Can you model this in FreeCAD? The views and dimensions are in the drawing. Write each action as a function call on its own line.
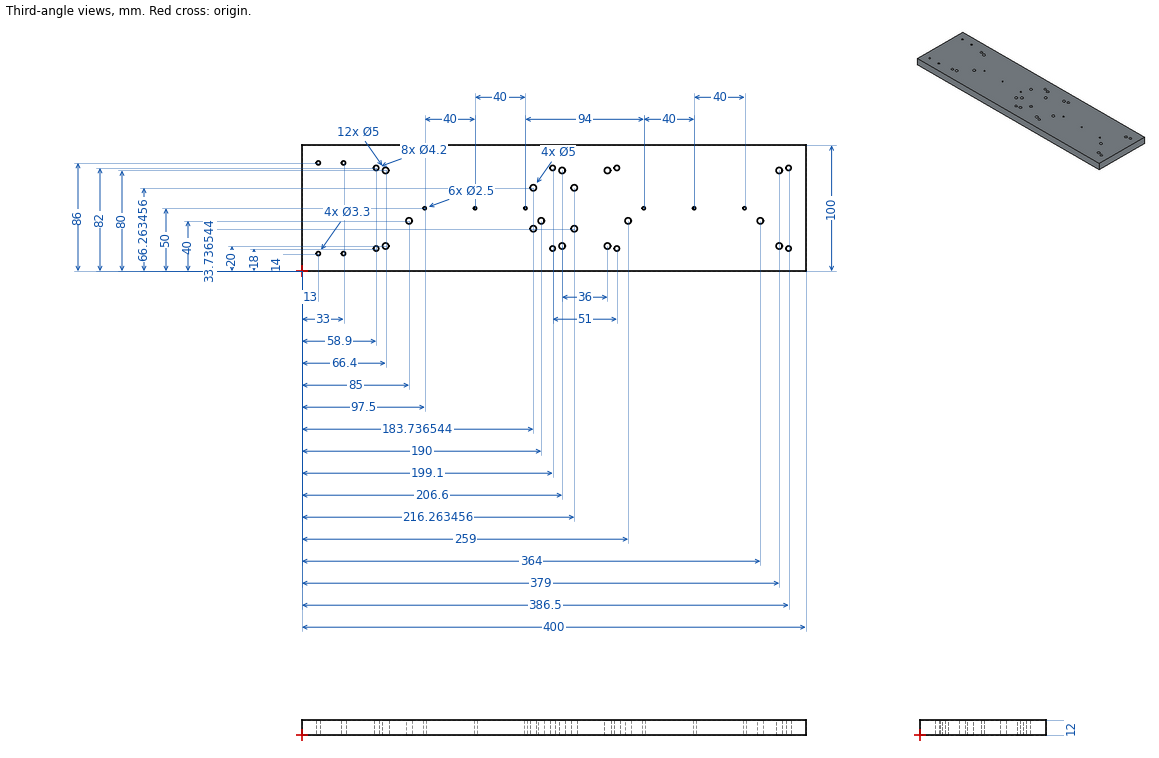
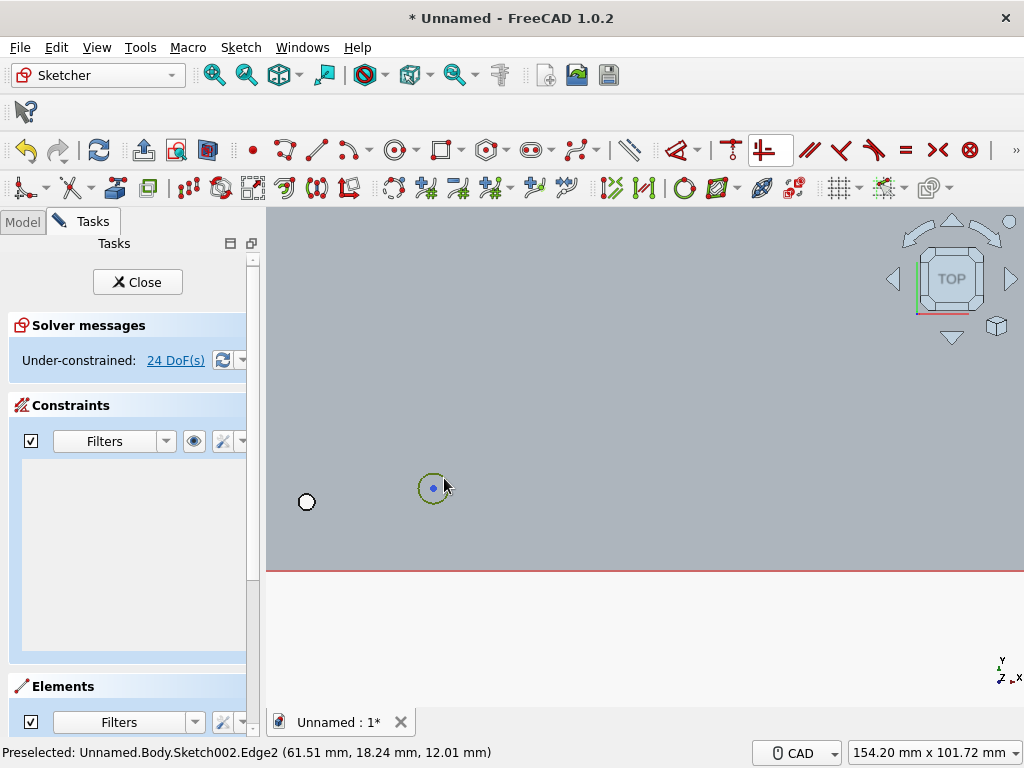
scroll(444, 480, down, 8)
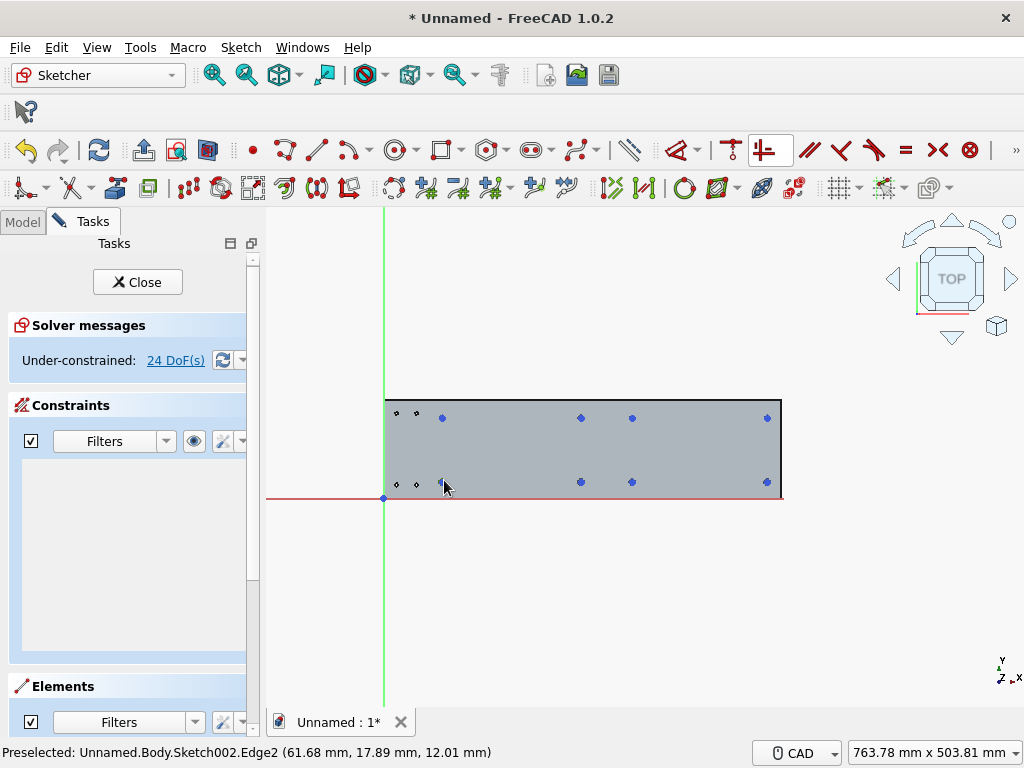
scroll(583, 416, up, 9)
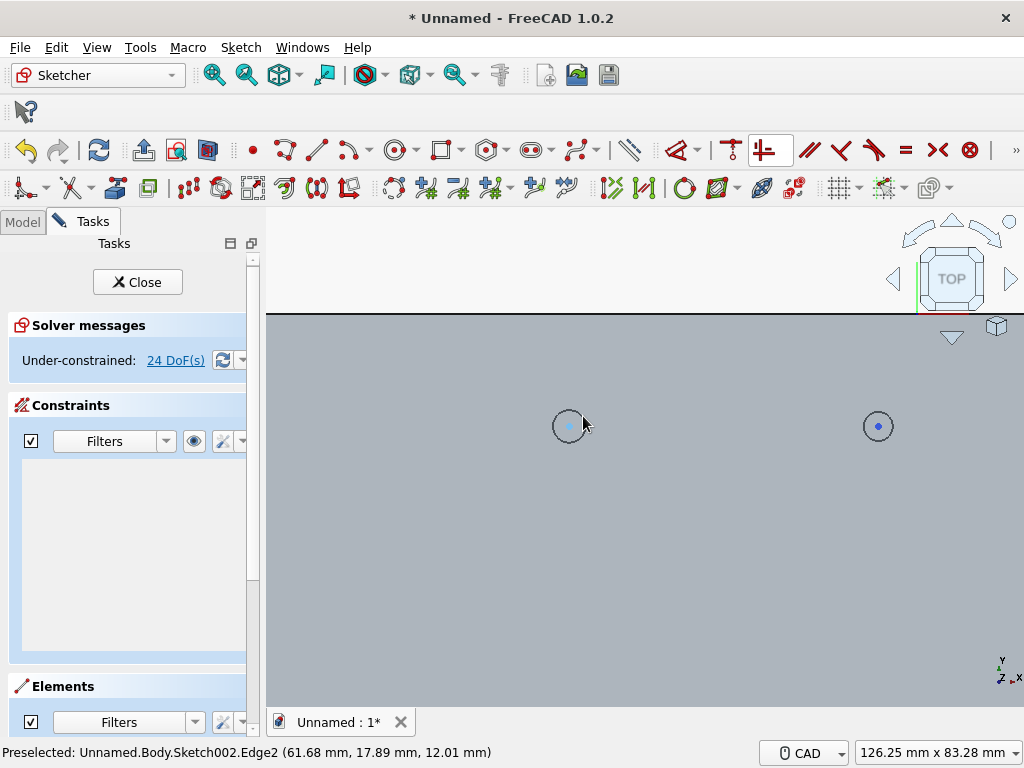
click(581, 415)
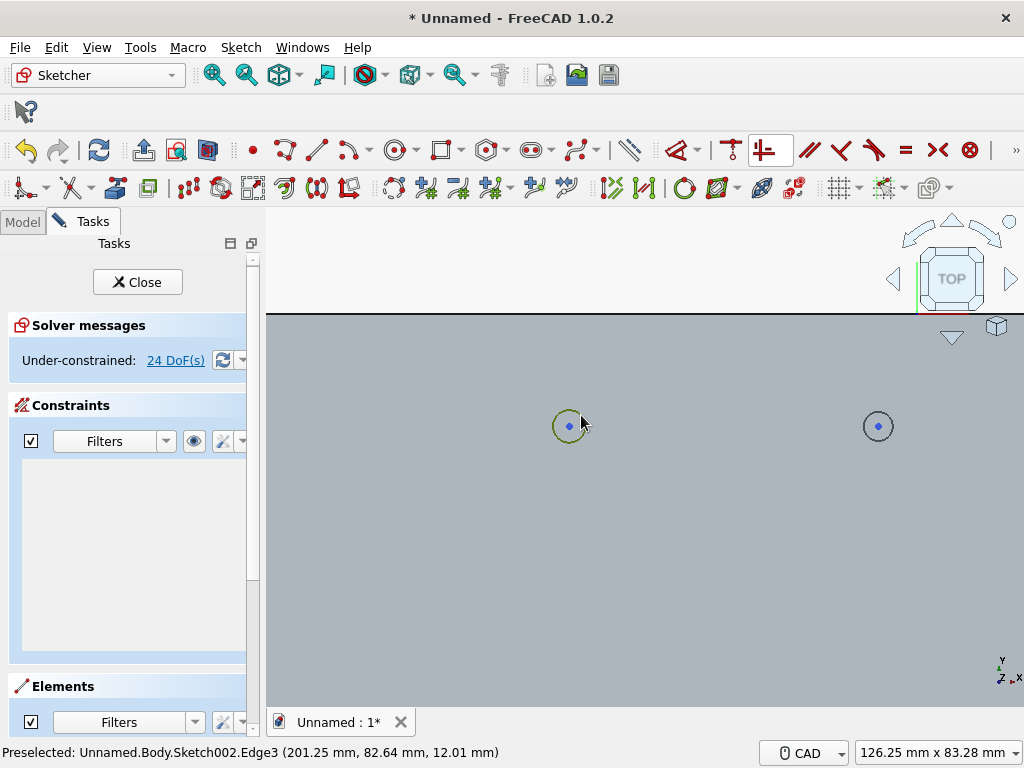
scroll(583, 416, down, 9)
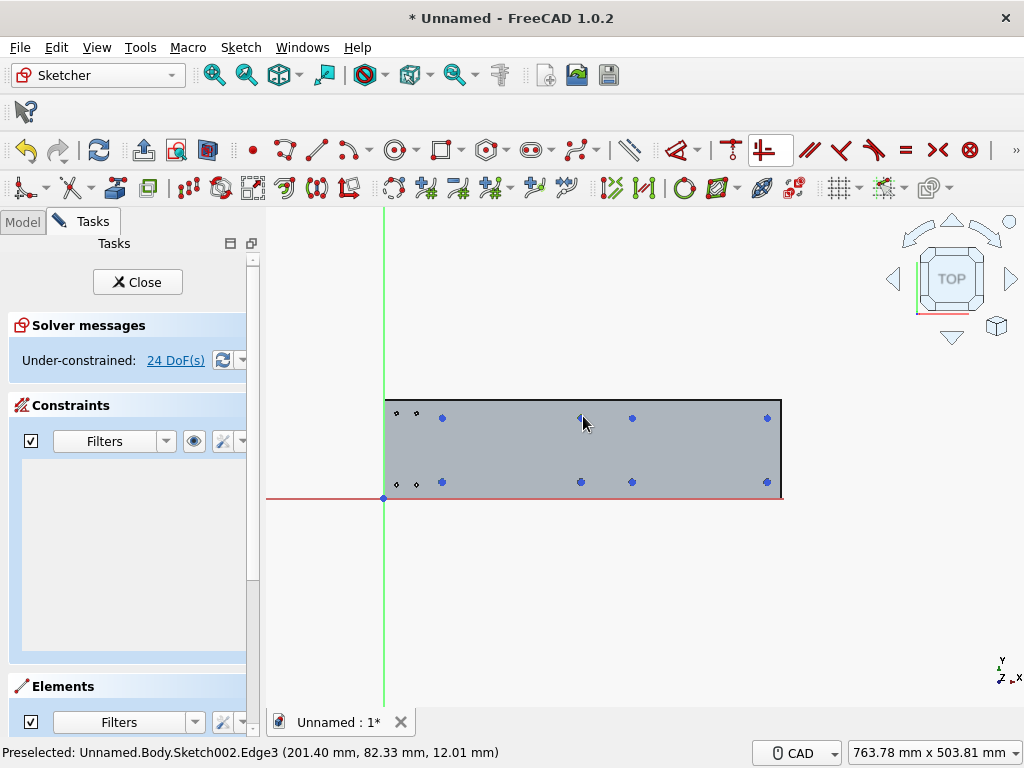
scroll(583, 480, up, 8)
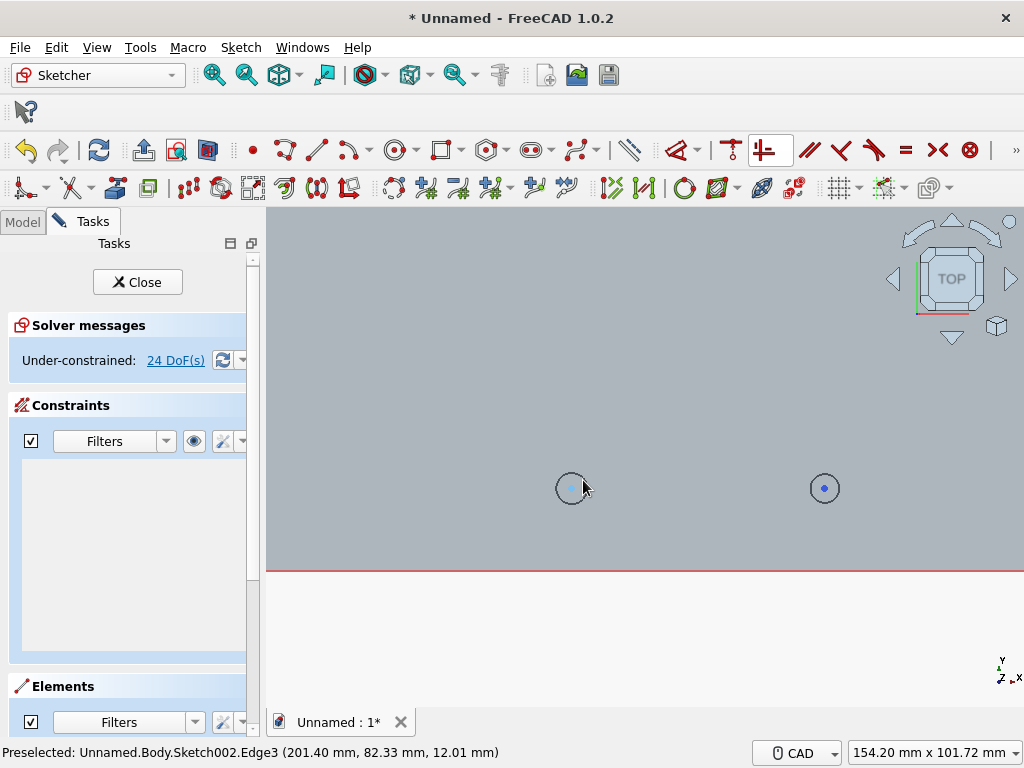
click(583, 478)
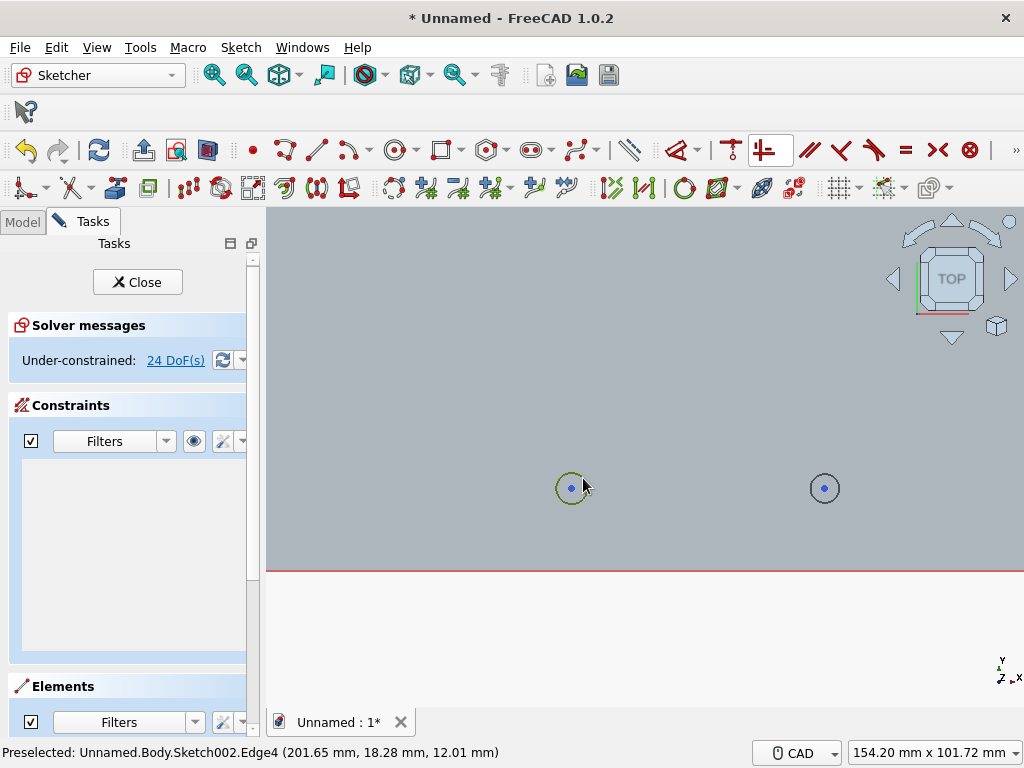
click(835, 478)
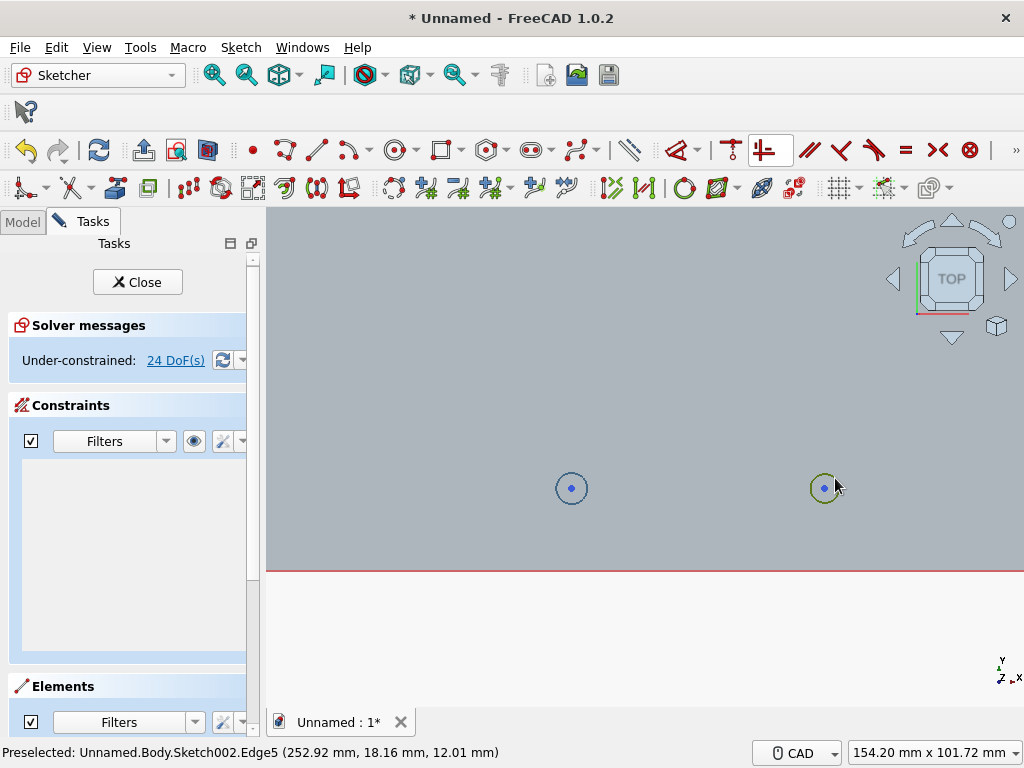
scroll(583, 480, down, 8)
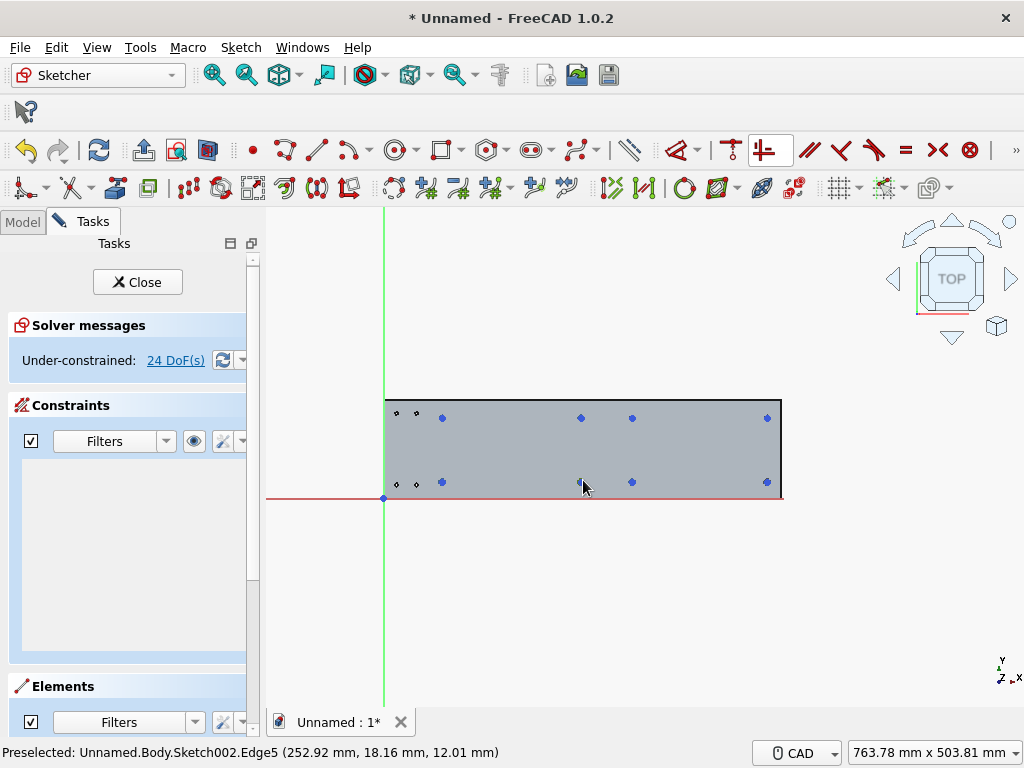
scroll(634, 416, up, 9)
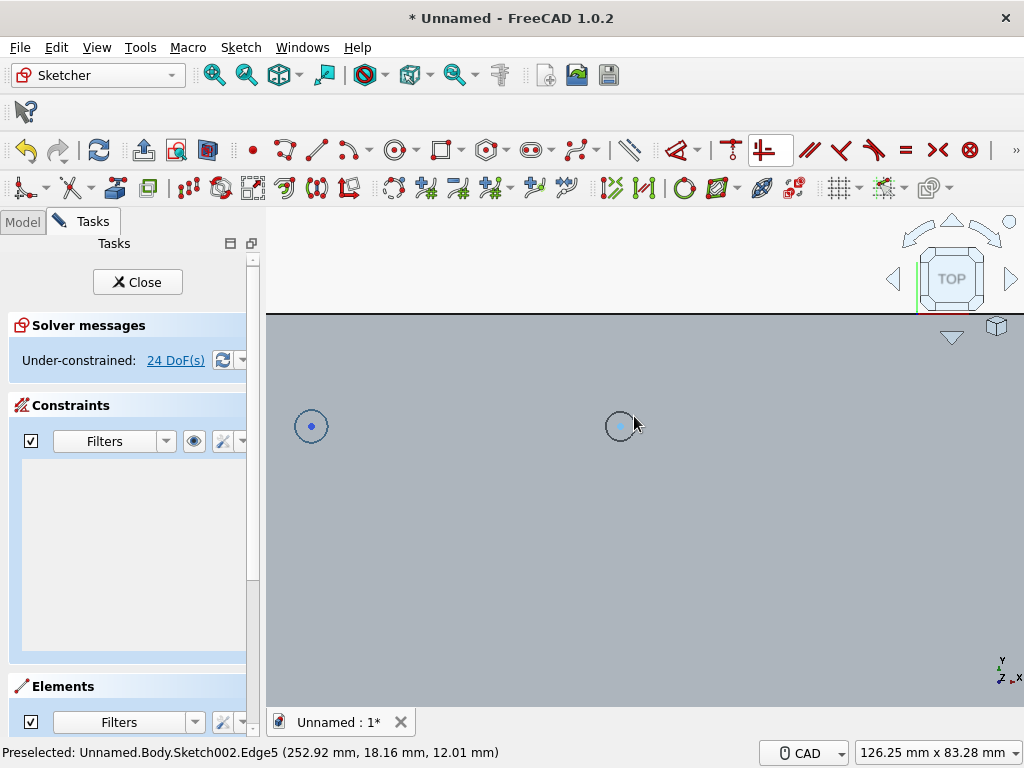
click(631, 416)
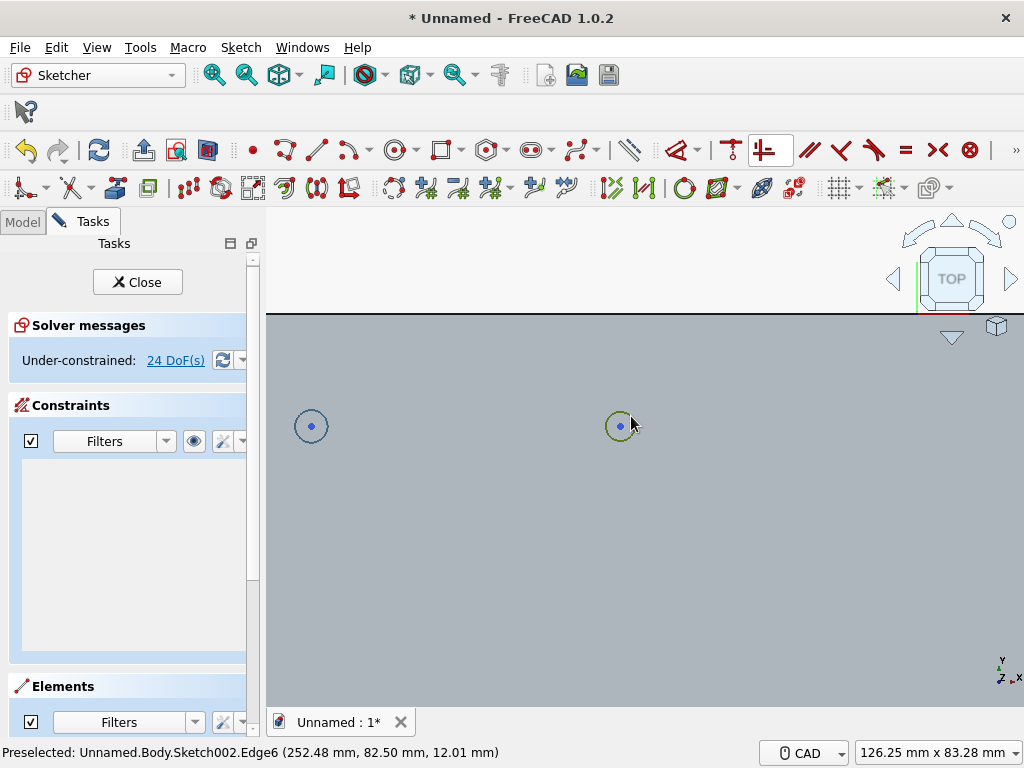
scroll(634, 416, down, 9)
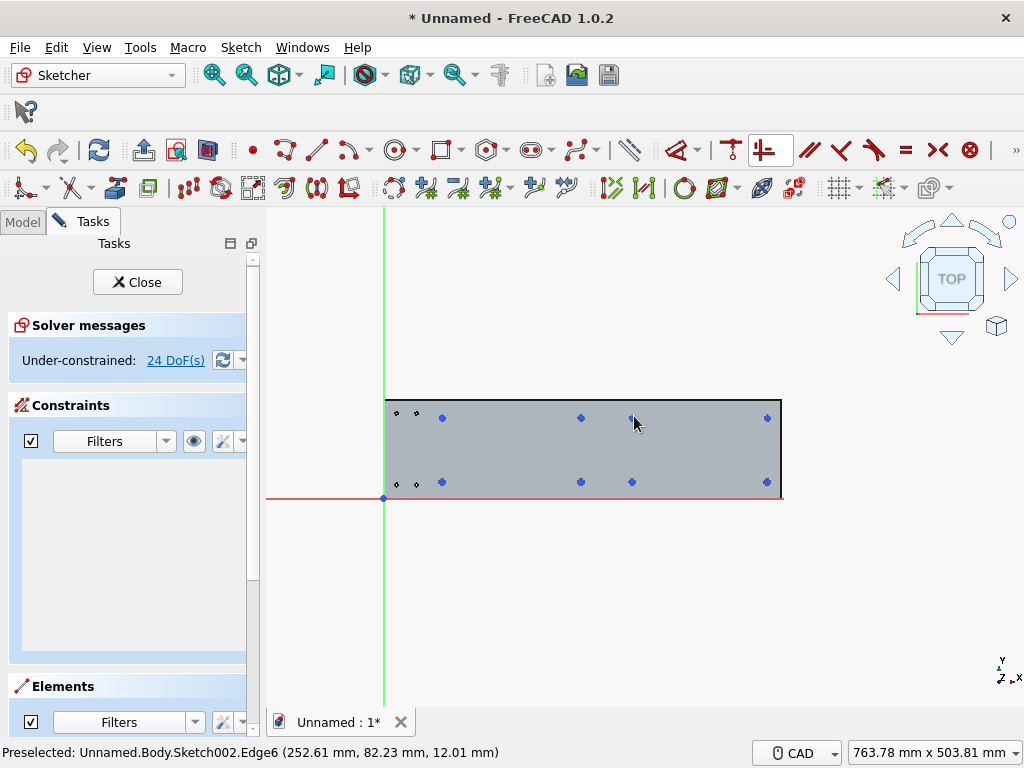
scroll(769, 416, up, 9)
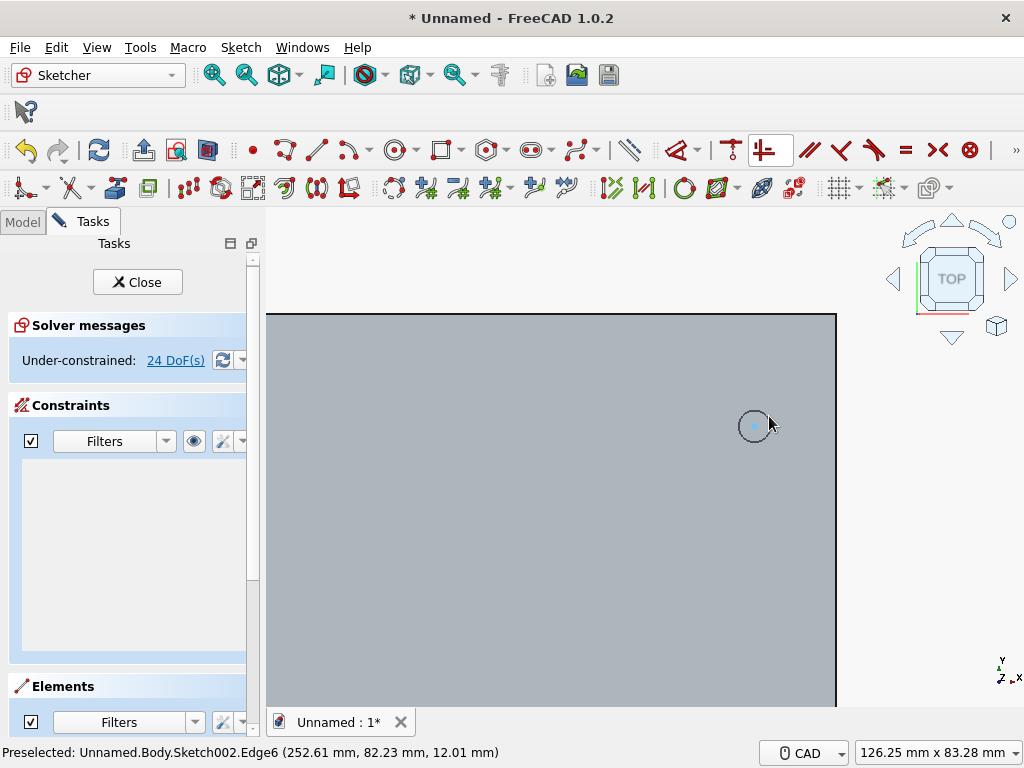
click(766, 415)